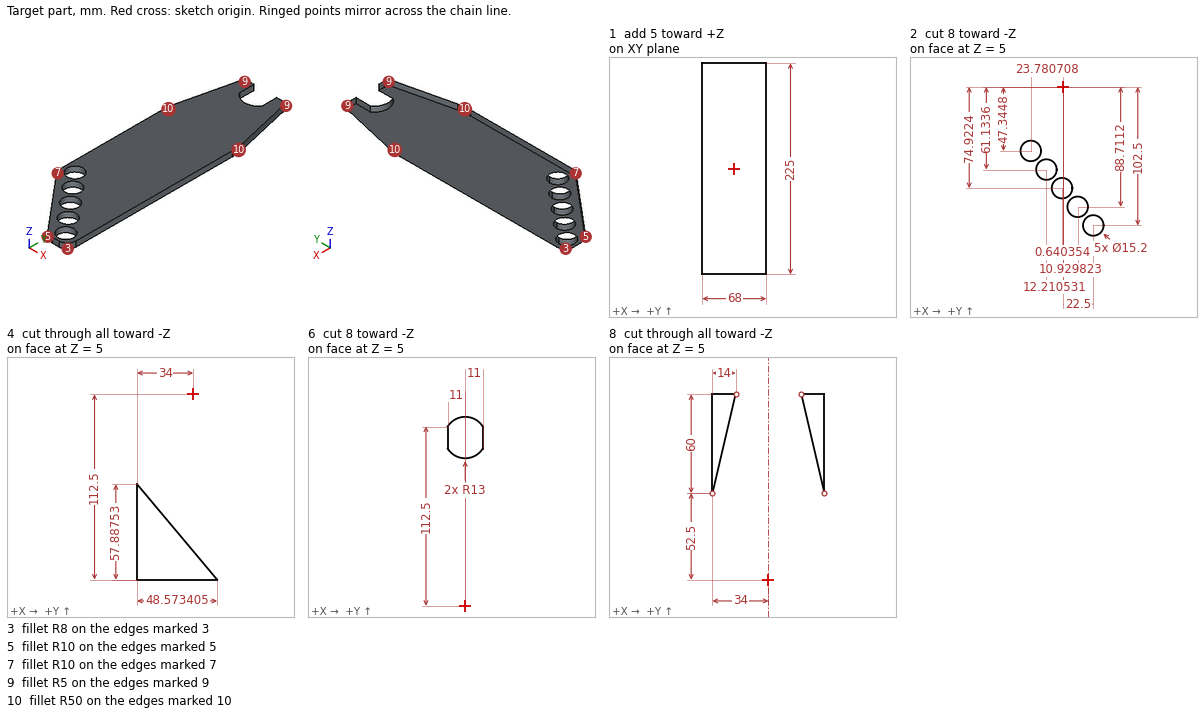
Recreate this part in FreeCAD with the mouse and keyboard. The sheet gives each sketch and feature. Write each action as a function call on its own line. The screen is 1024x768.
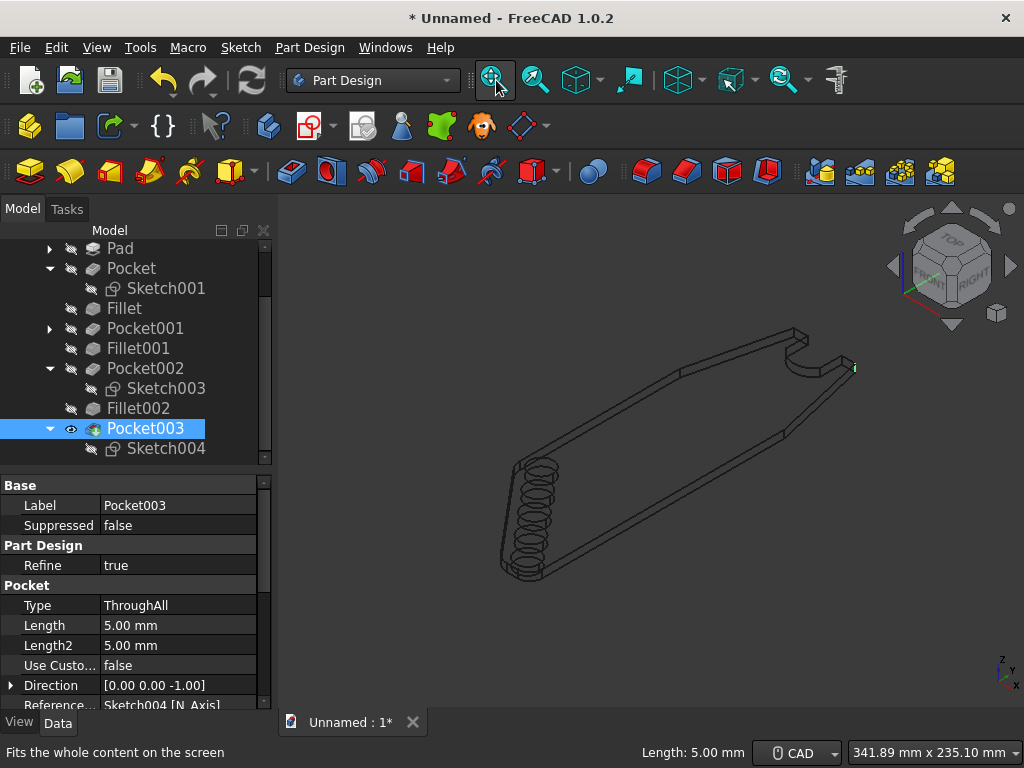
scroll(794, 331, up, 7)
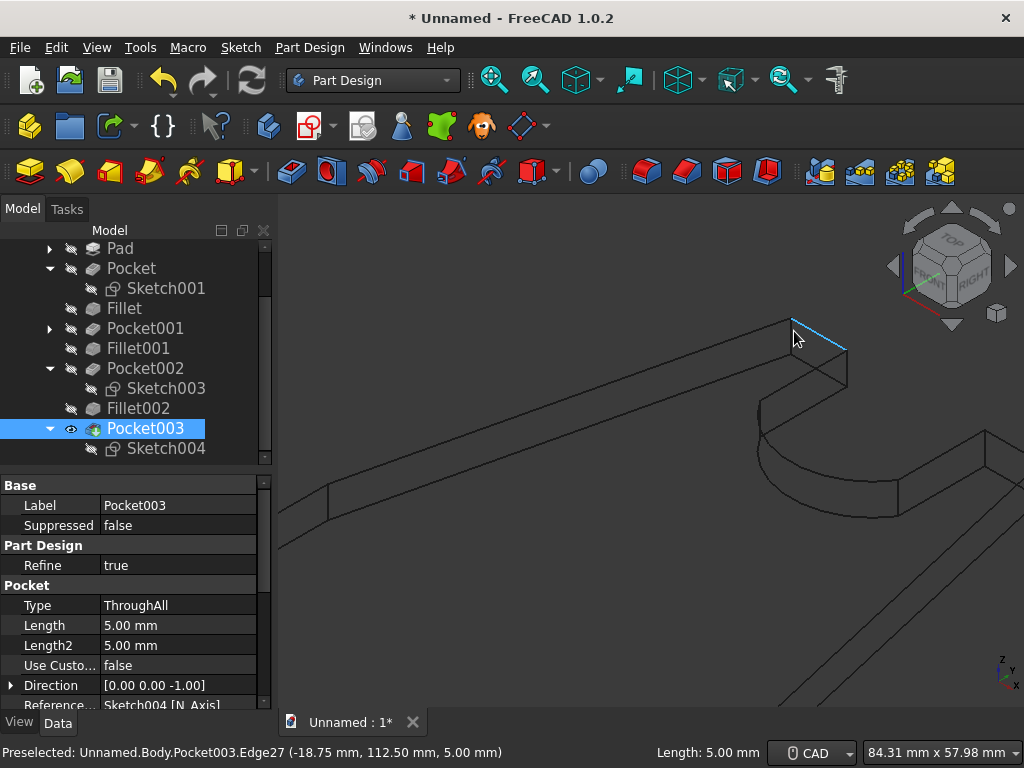
click(791, 335, ctrl)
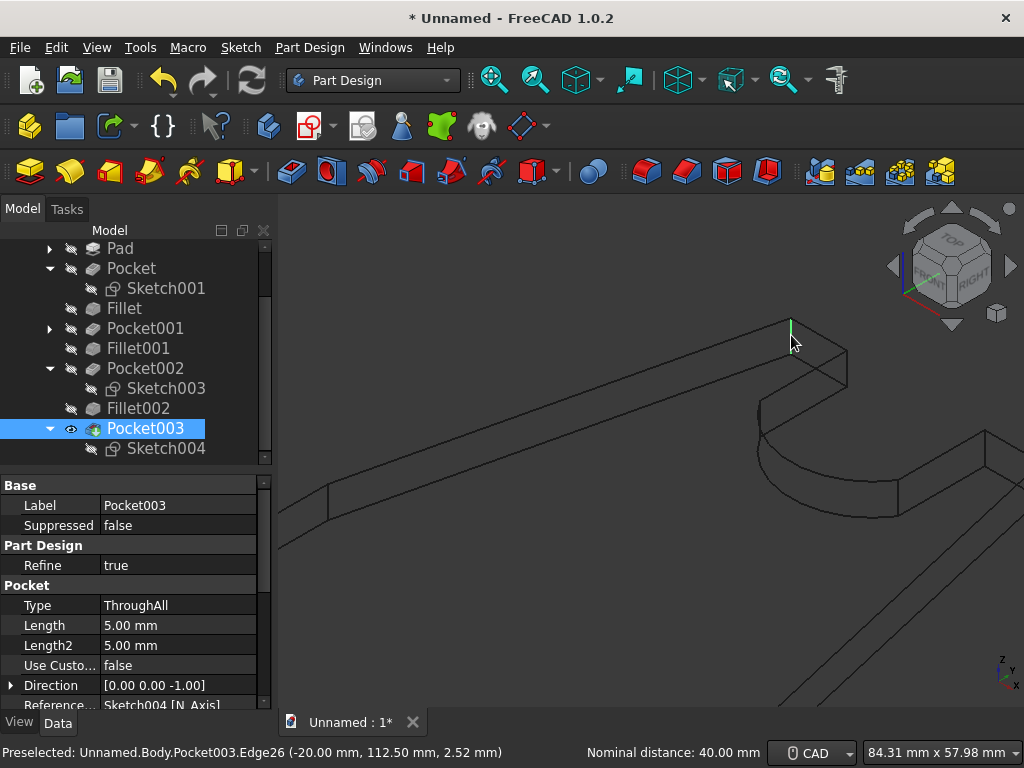
key(v)
key(1)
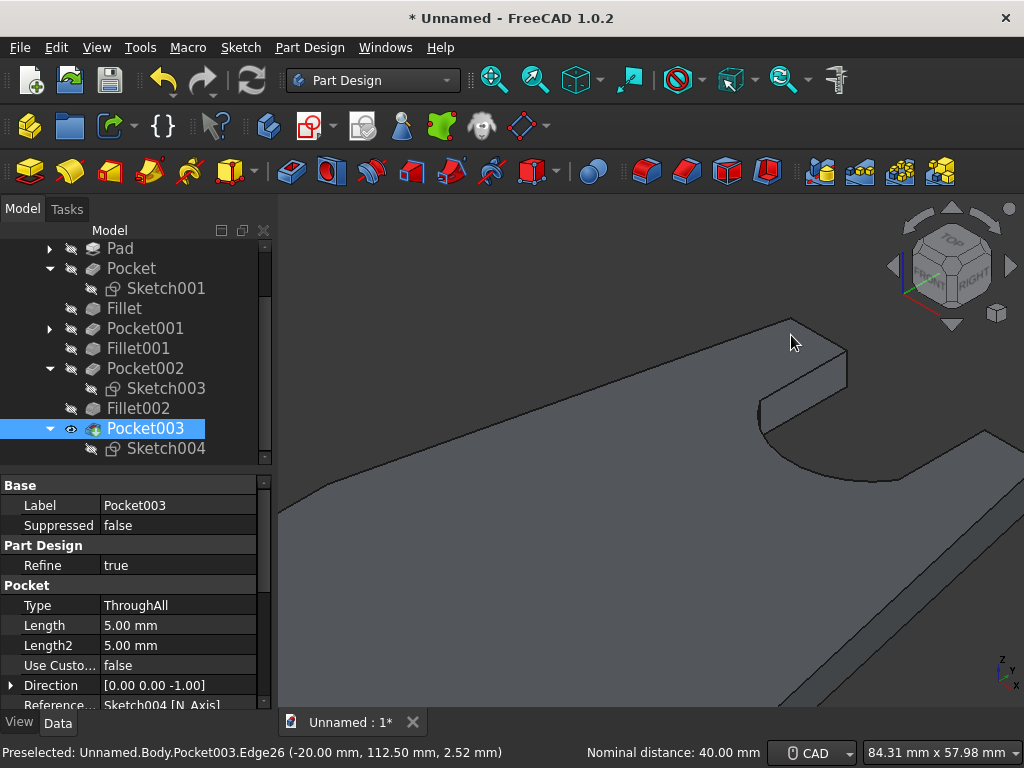
click(648, 172)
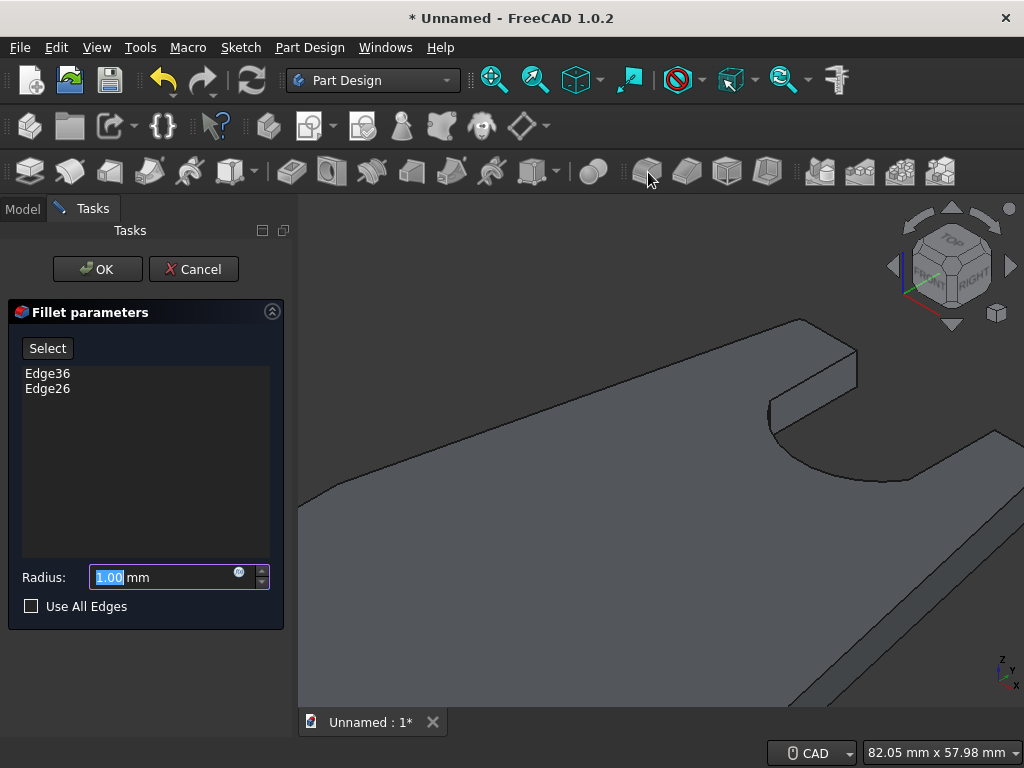
text(5)
key(Tab)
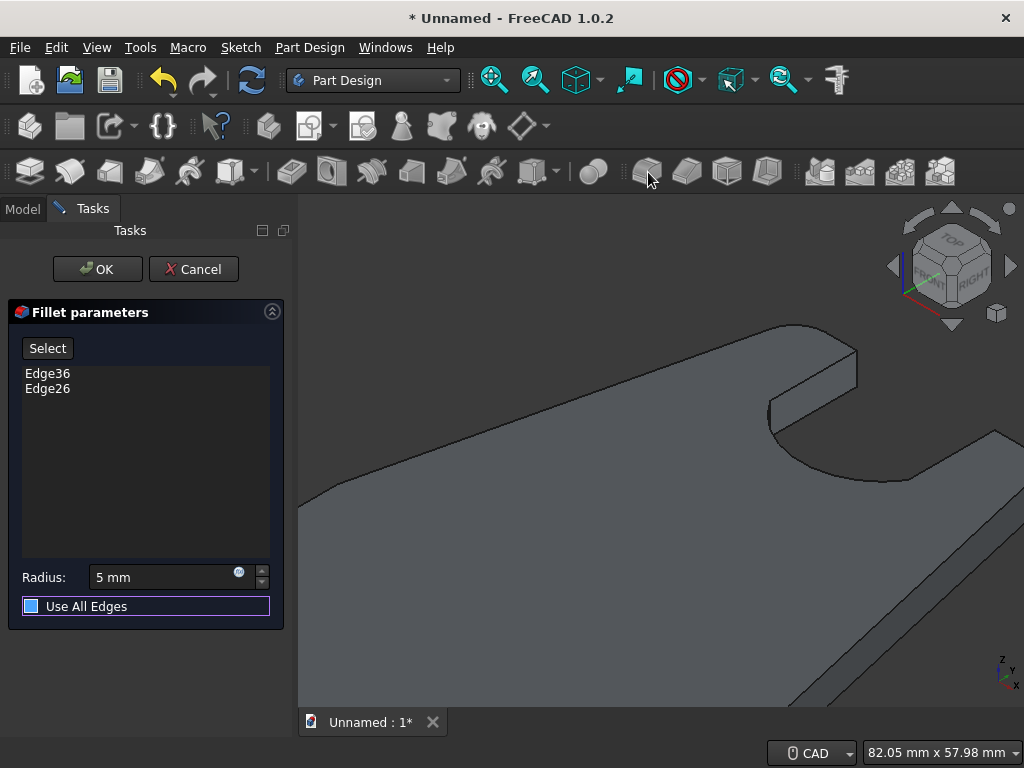
click(98, 269)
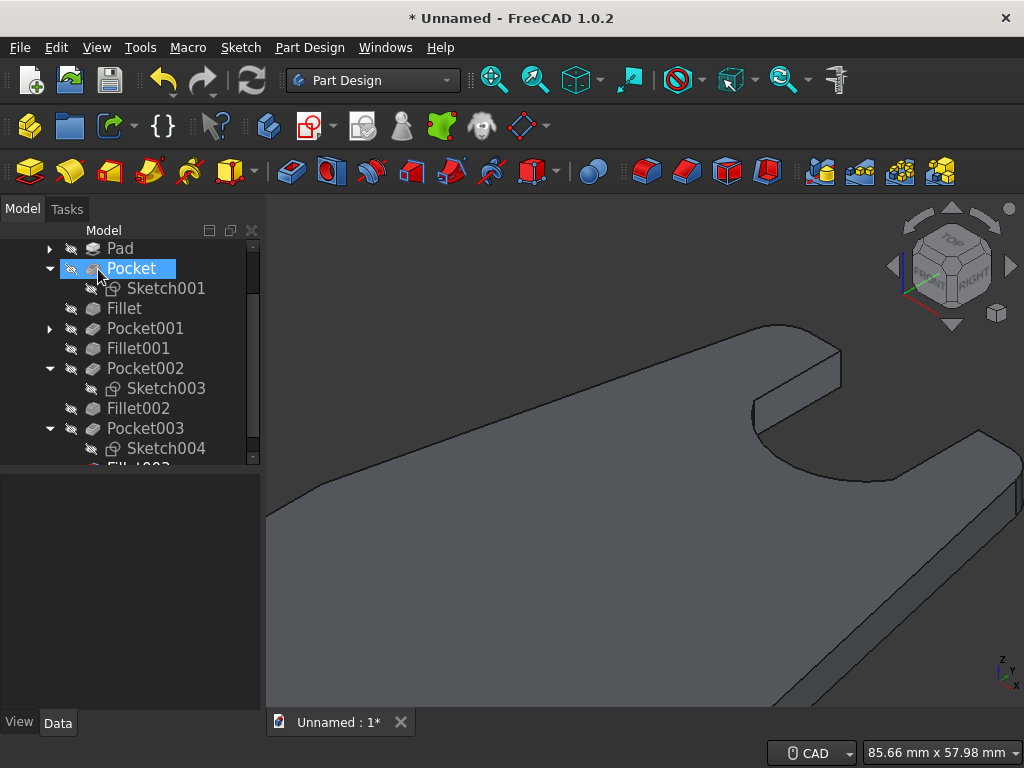
click(496, 80)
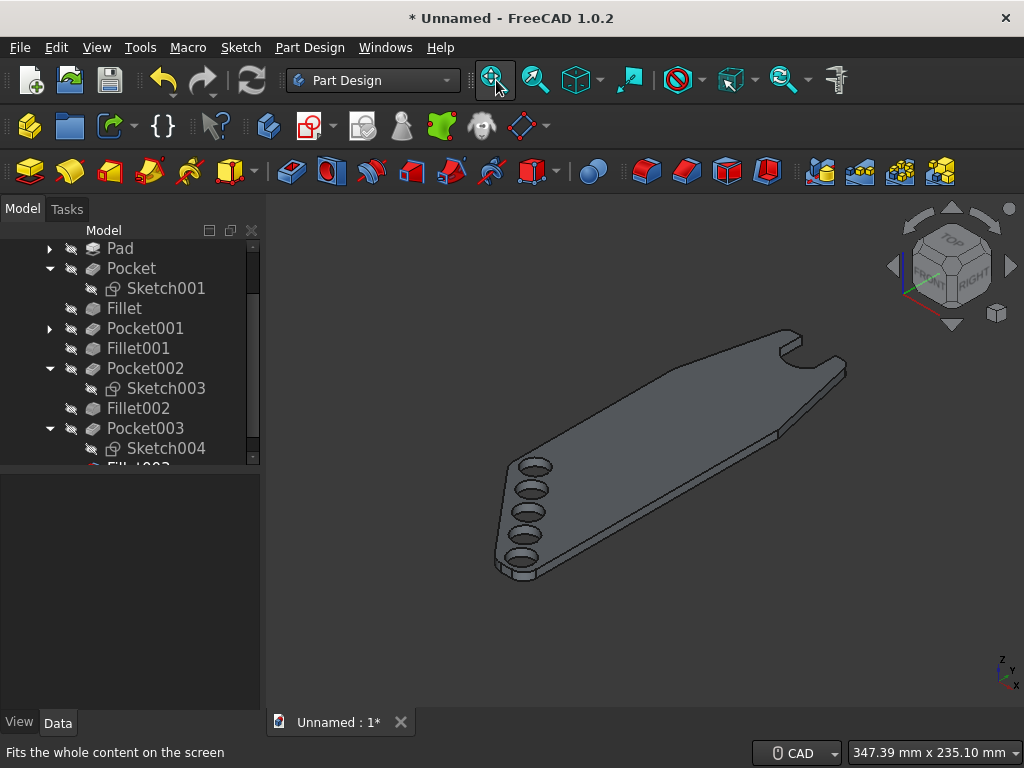
scroll(778, 433, up, 7)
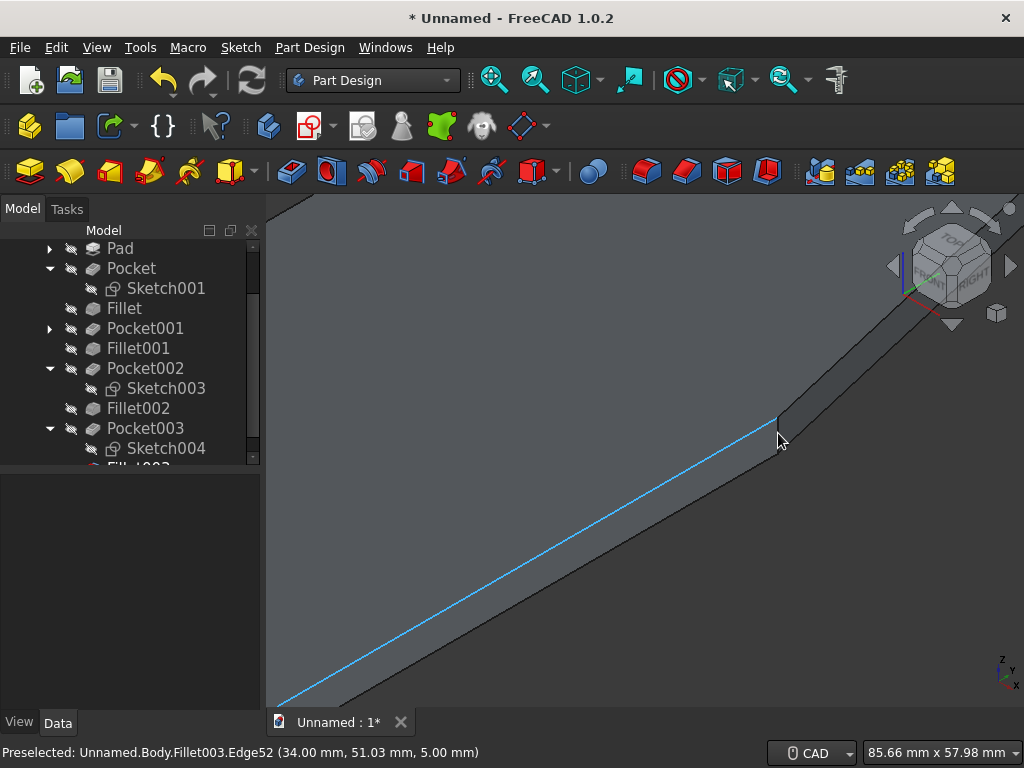
key(v)
key(f)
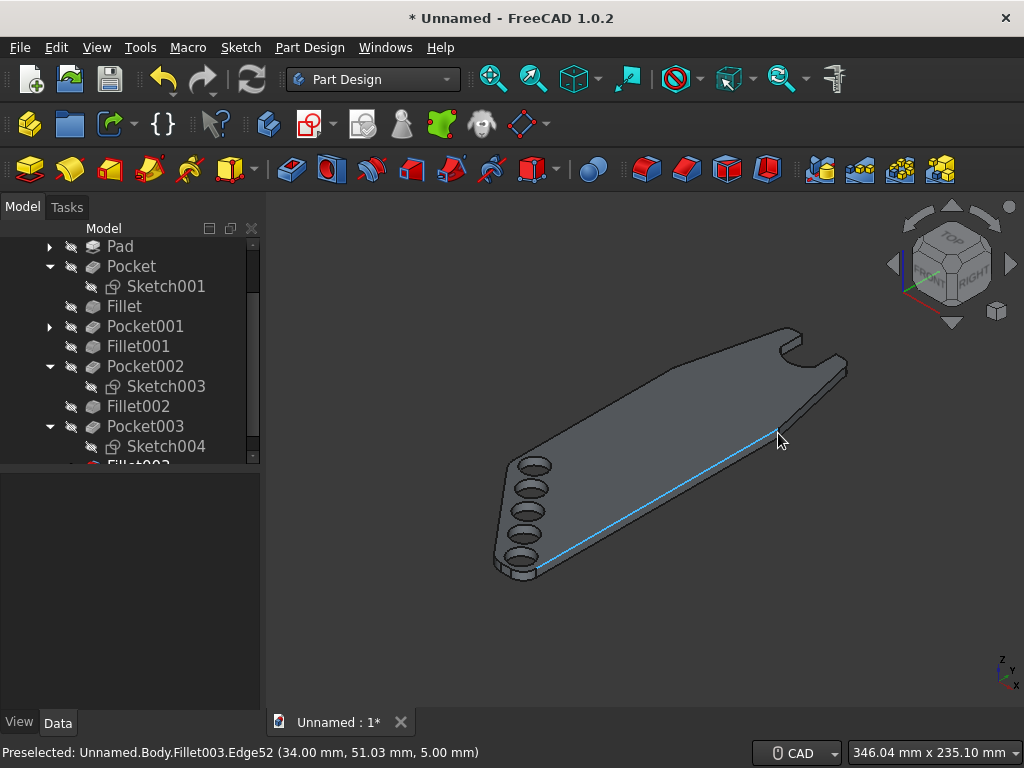
key(2)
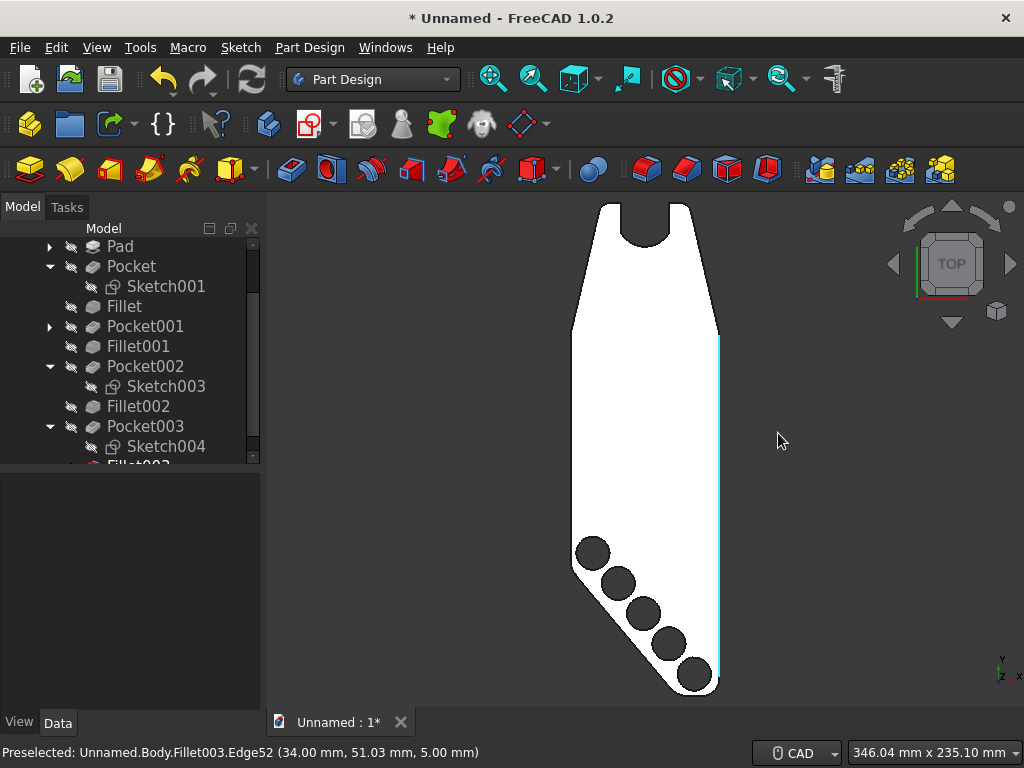
scroll(719, 333, up, 7)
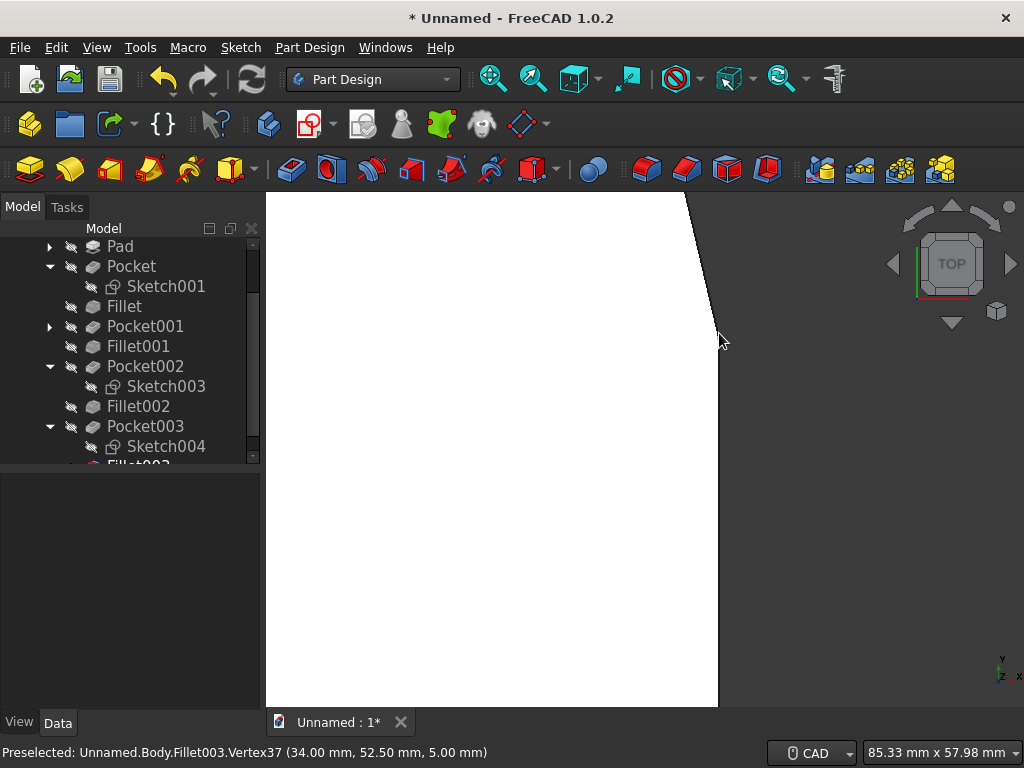
key(v)
key(f)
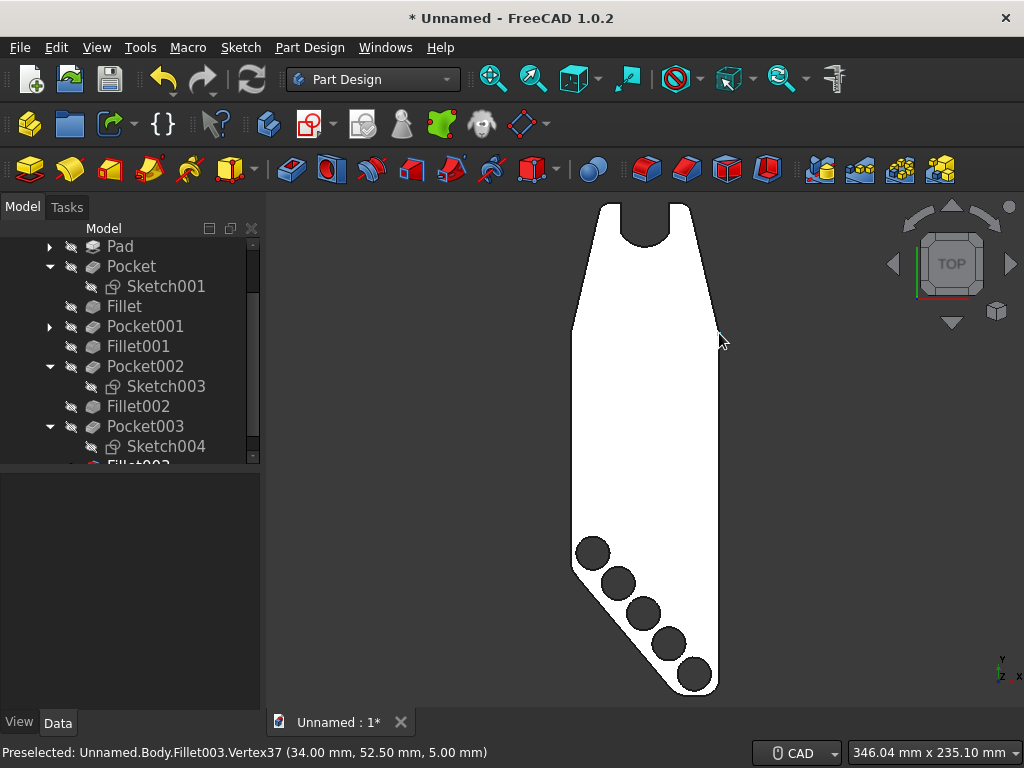
key(0)